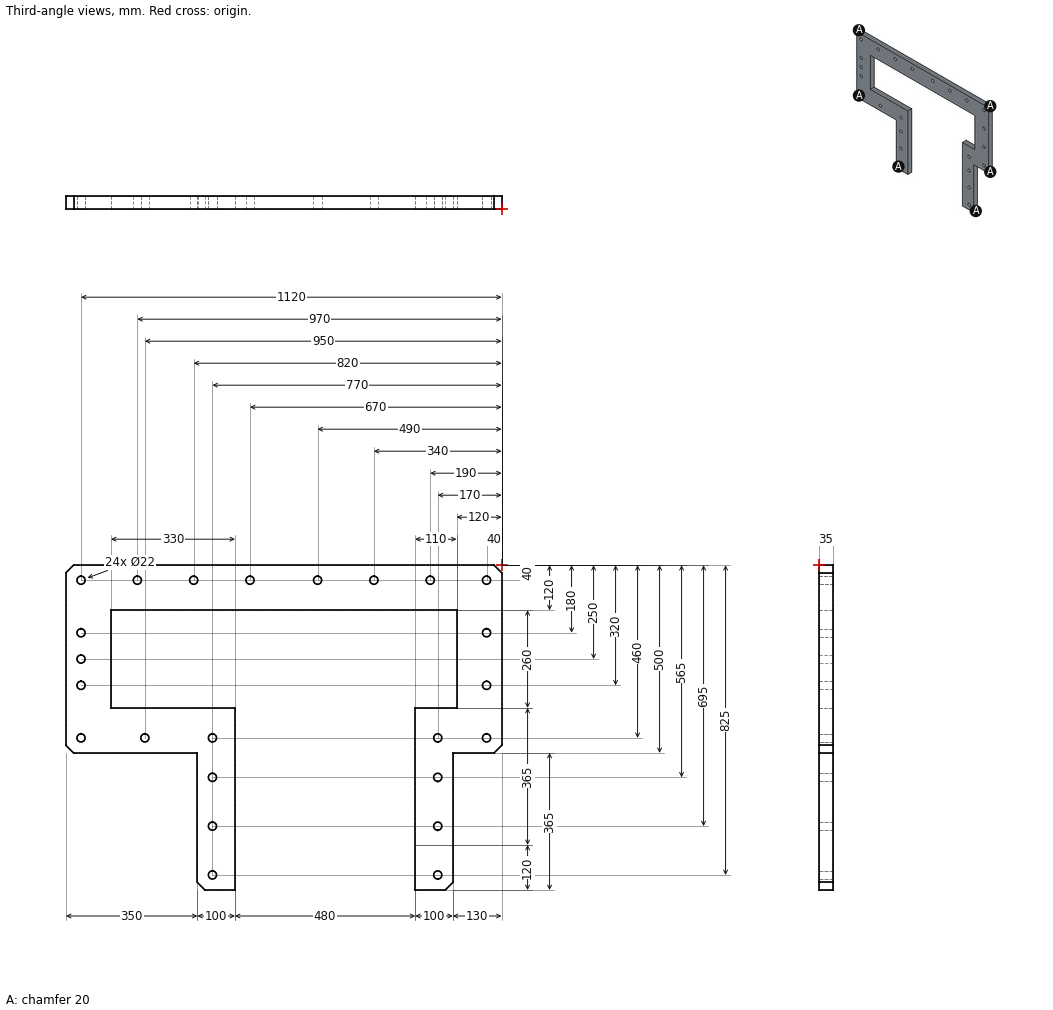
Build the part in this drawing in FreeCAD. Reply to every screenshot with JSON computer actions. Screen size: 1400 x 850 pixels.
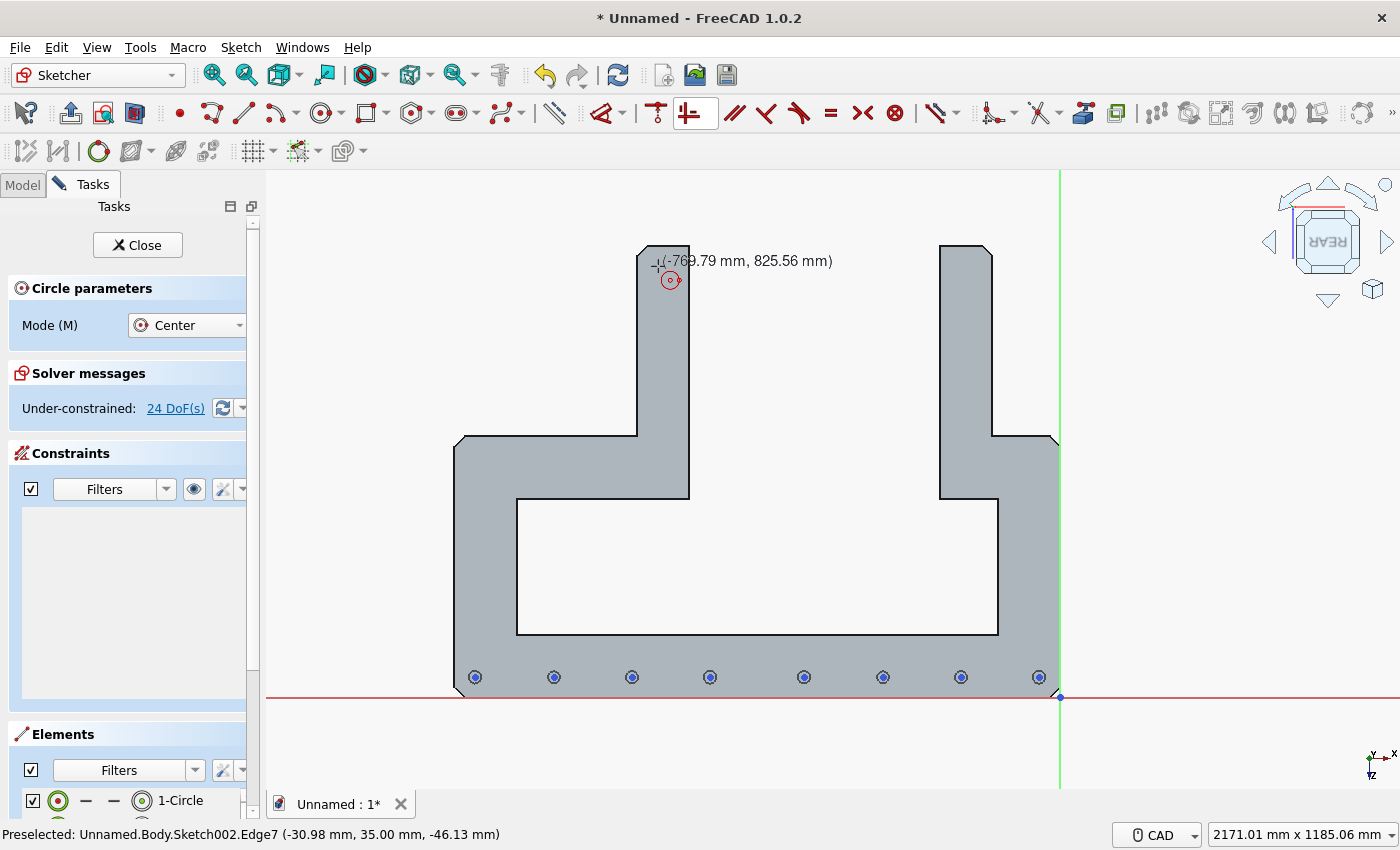
{"action": "left_click", "coordinate": [658, 267]}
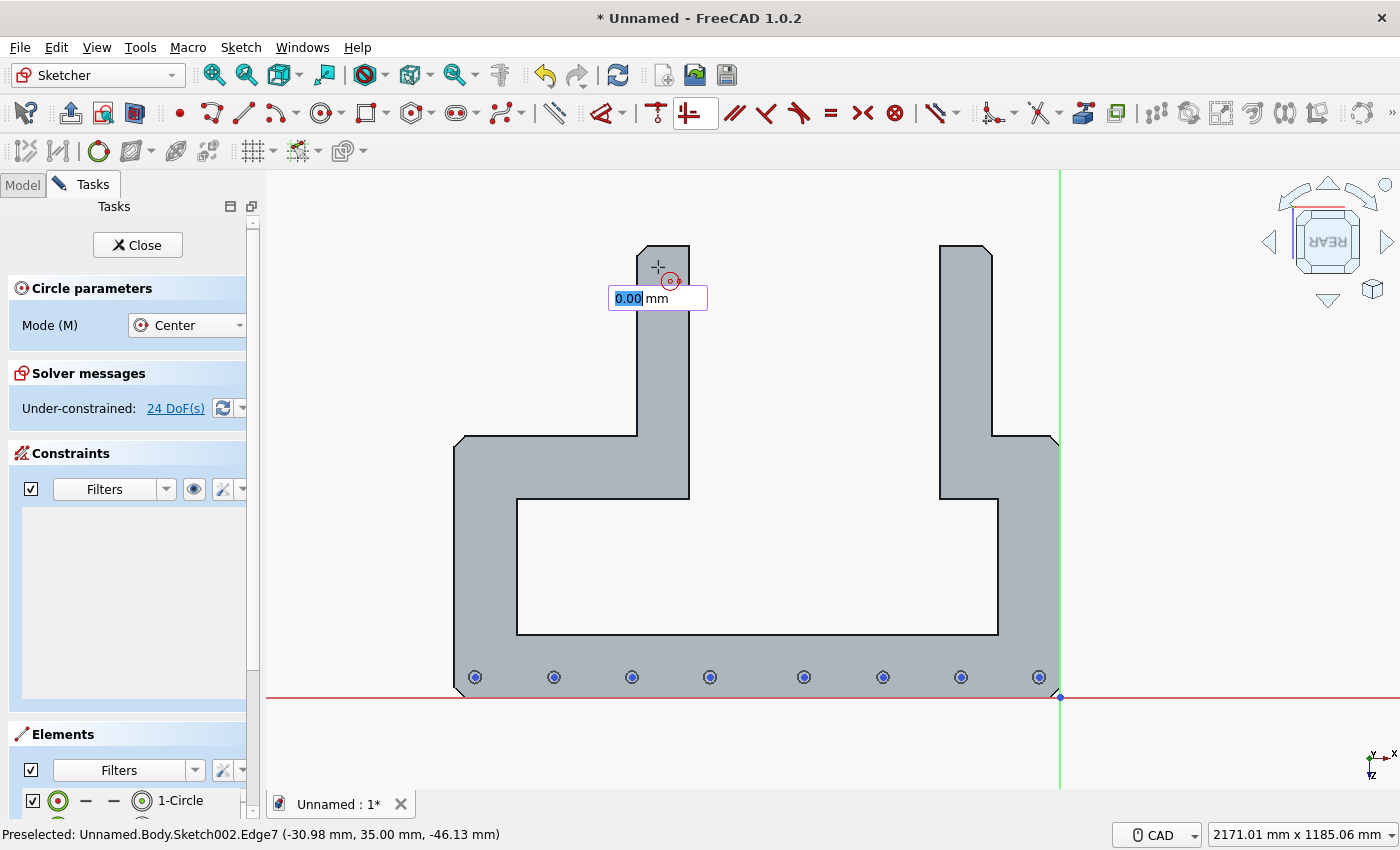
{"action": "scroll", "coordinate": [662, 263], "scroll_direction": "up", "scroll_amount": 6}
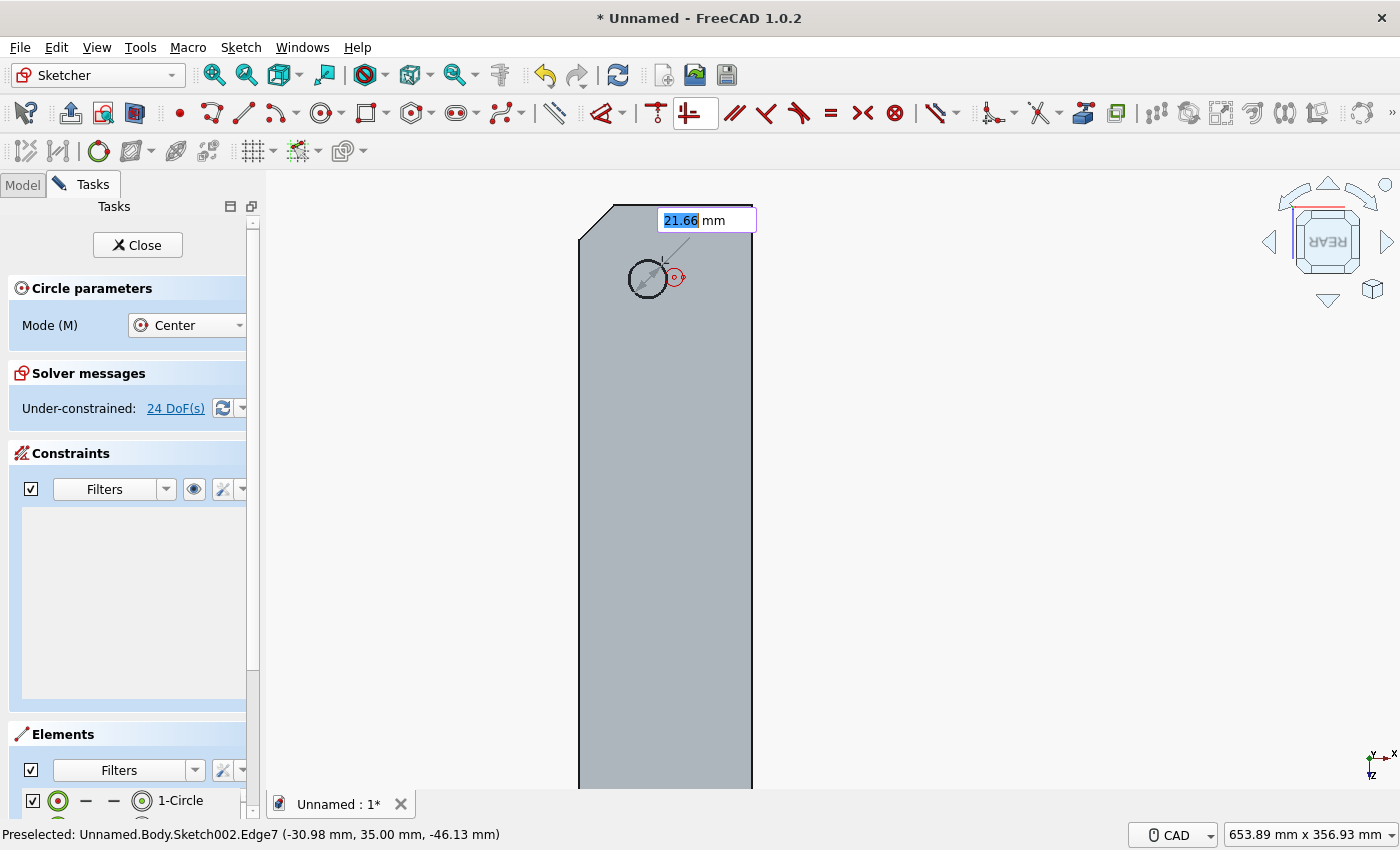
{"action": "left_click", "coordinate": [662, 261]}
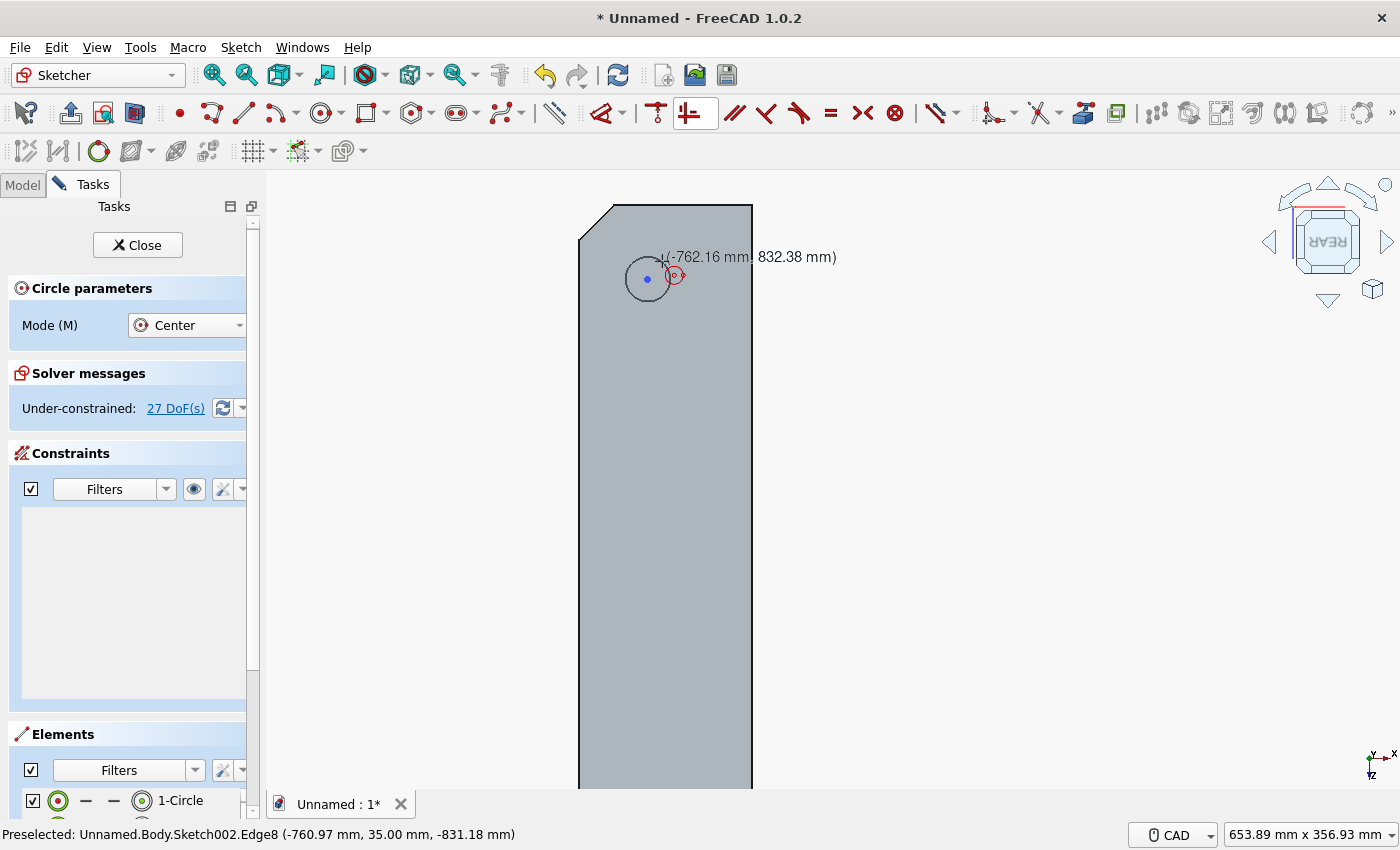
{"action": "scroll", "coordinate": [662, 264], "scroll_direction": "down", "scroll_amount": 6}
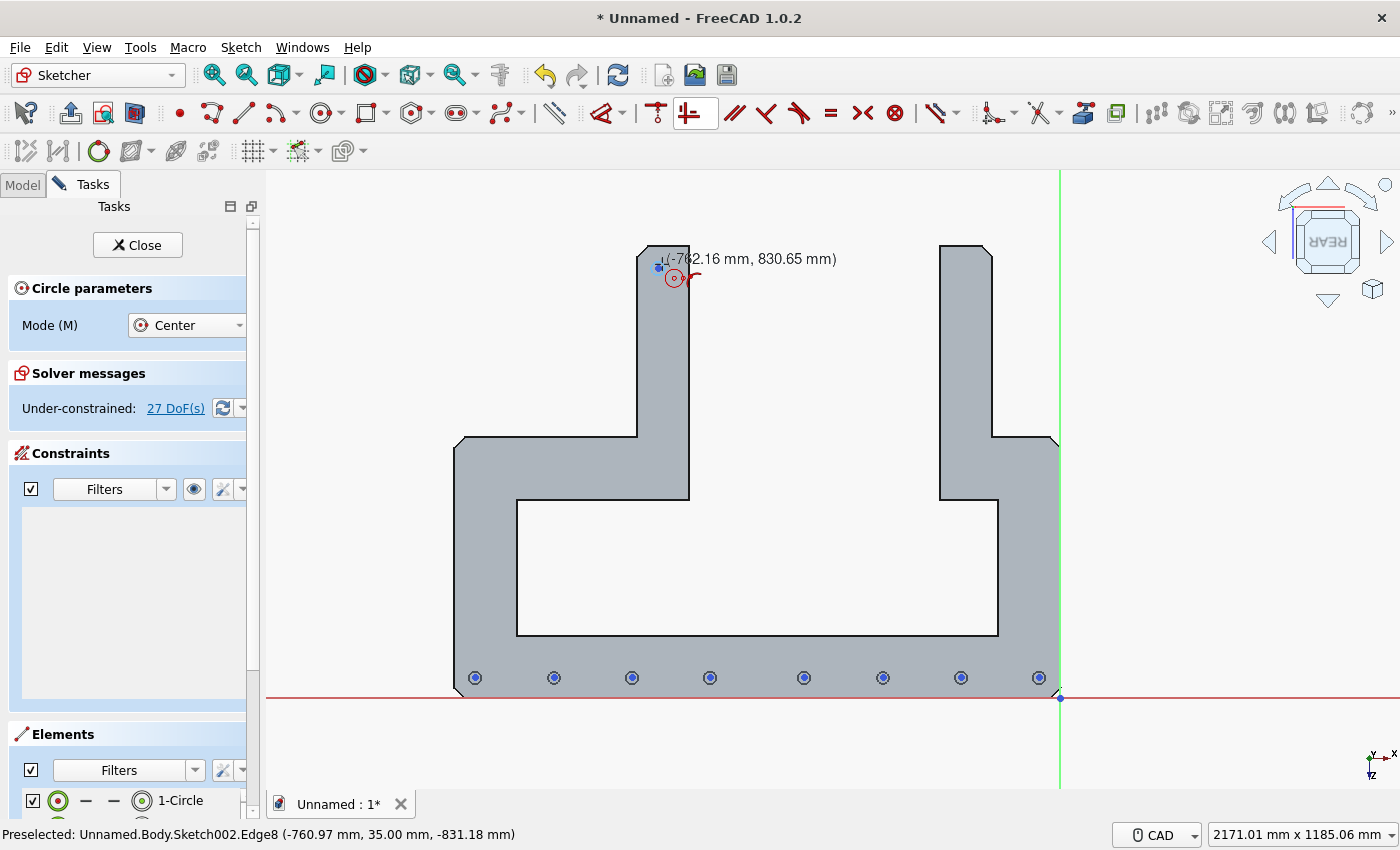
{"action": "left_click", "coordinate": [658, 335]}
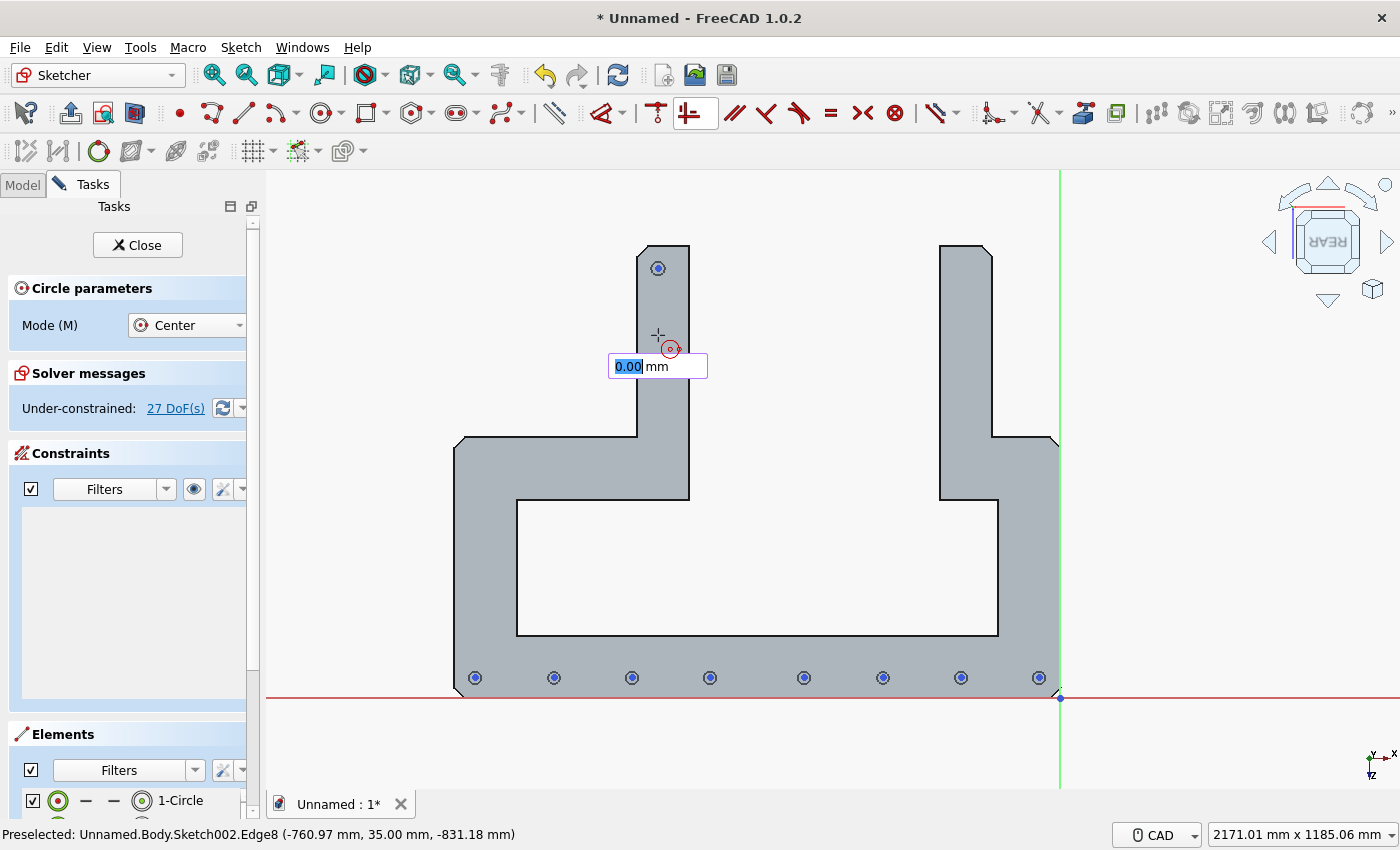
{"action": "scroll", "coordinate": [662, 331], "scroll_direction": "up", "scroll_amount": 6}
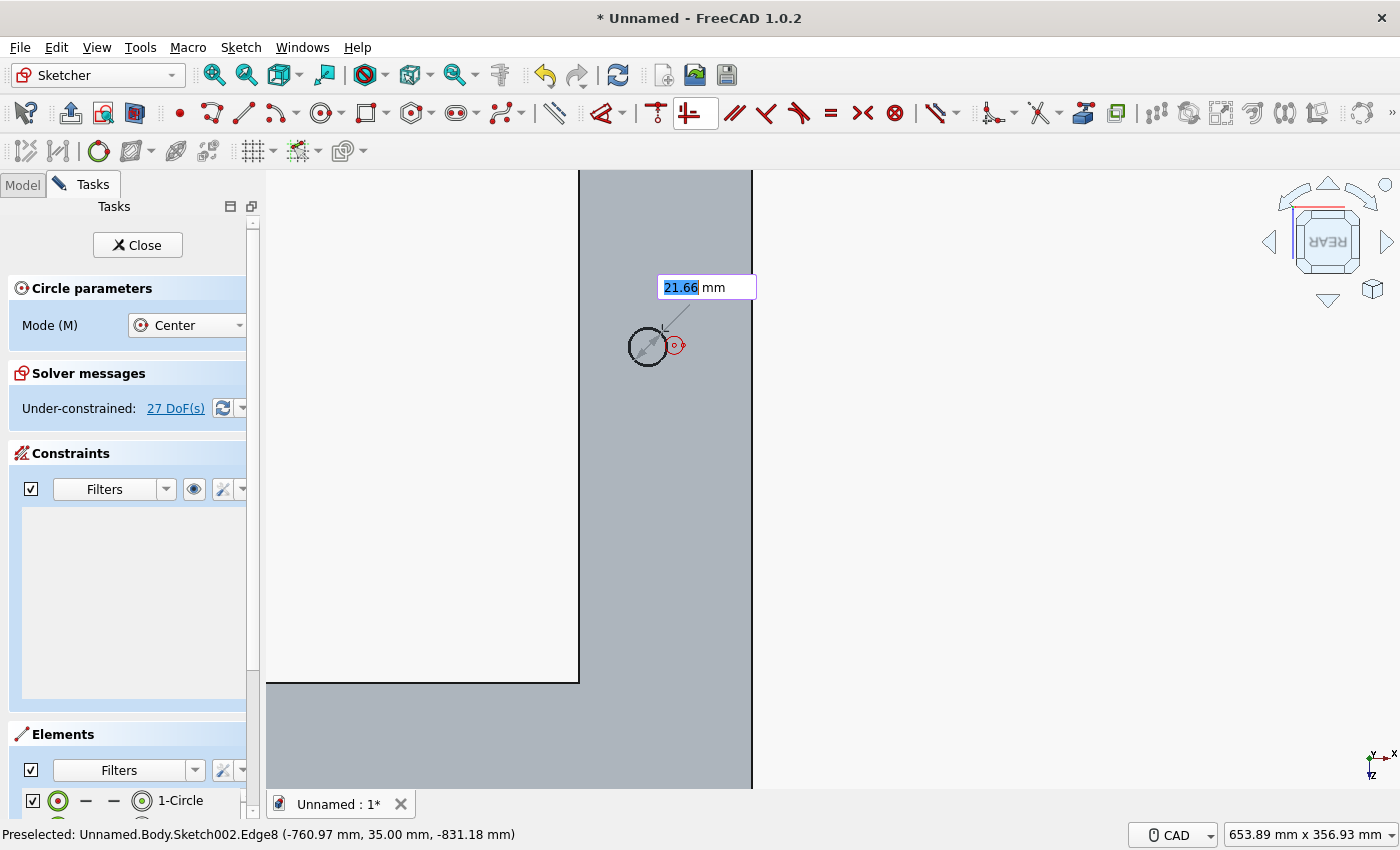
{"action": "left_click", "coordinate": [662, 331]}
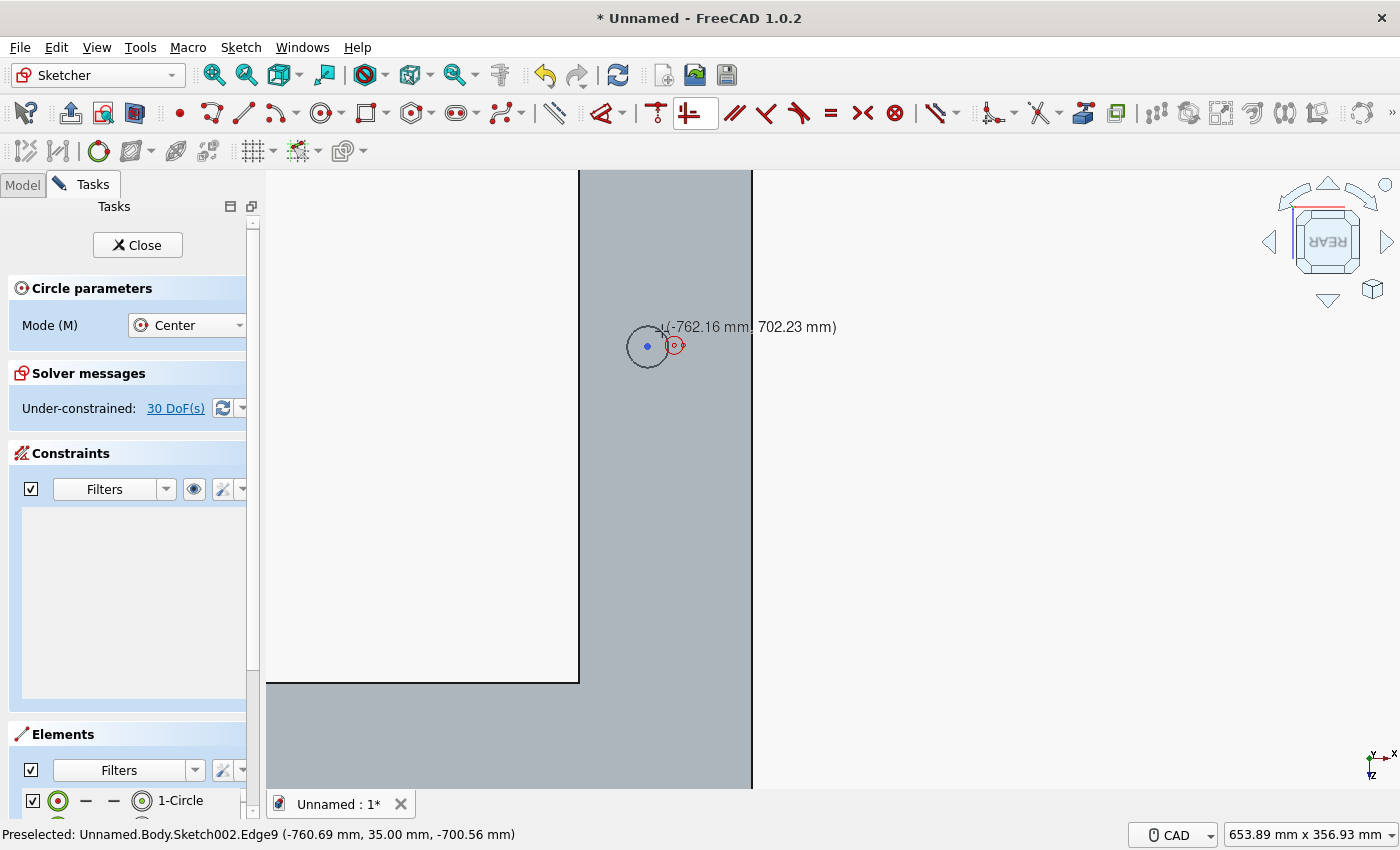
{"action": "scroll", "coordinate": [662, 331], "scroll_direction": "down", "scroll_amount": 6}